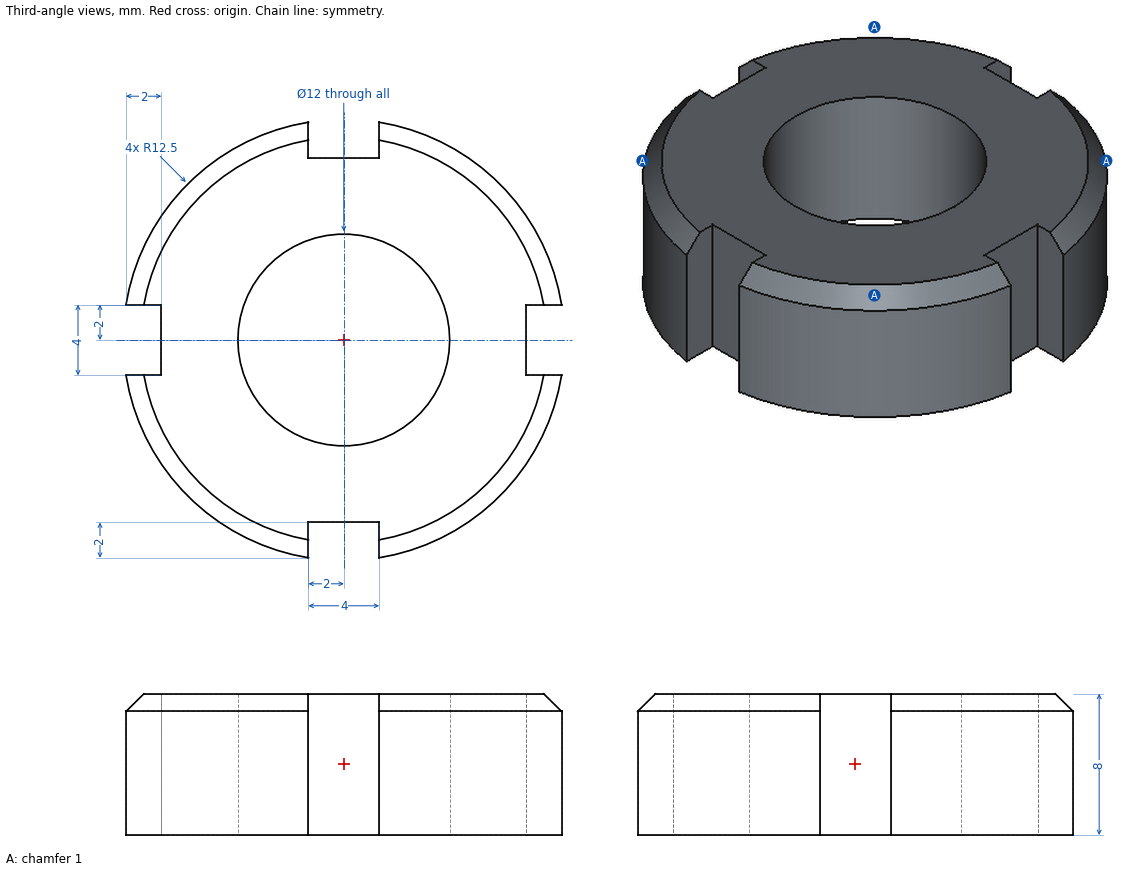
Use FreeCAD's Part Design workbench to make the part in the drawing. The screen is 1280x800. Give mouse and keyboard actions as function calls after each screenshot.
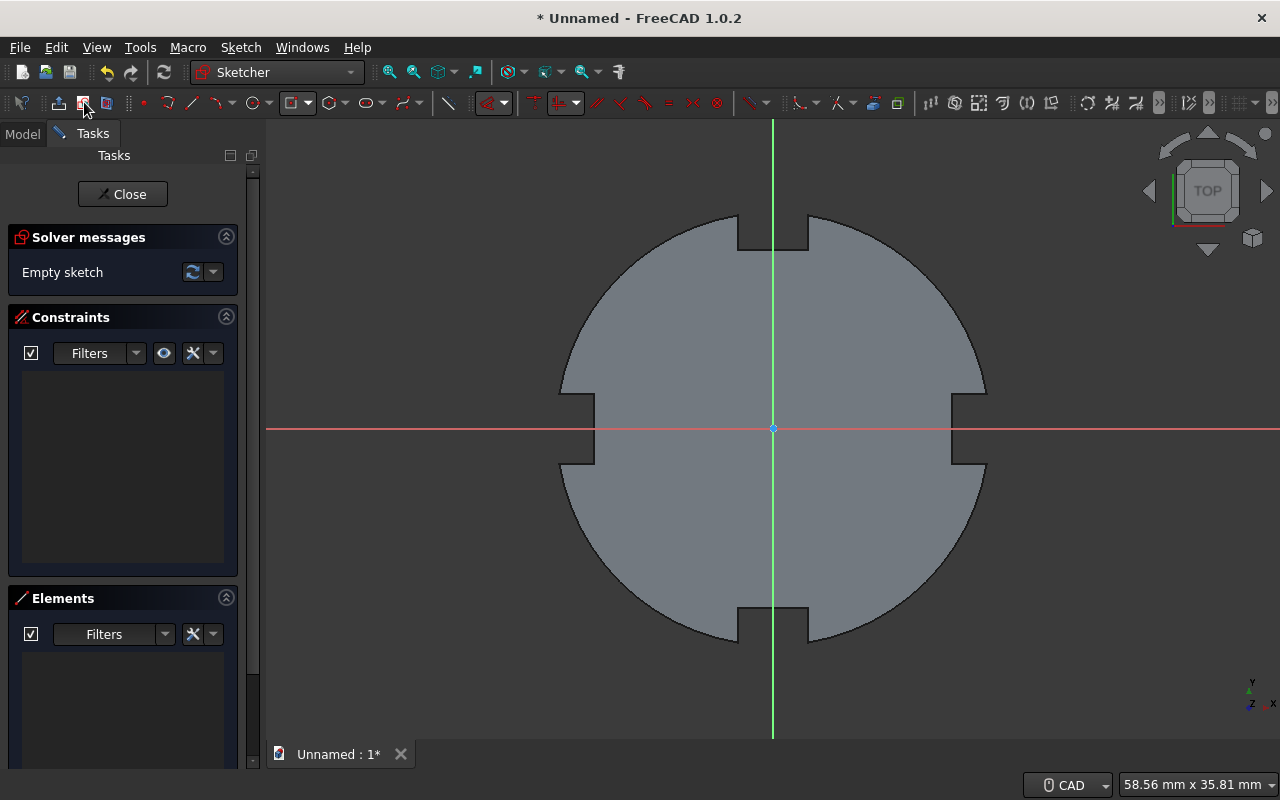
scroll(856, 429, up, 3)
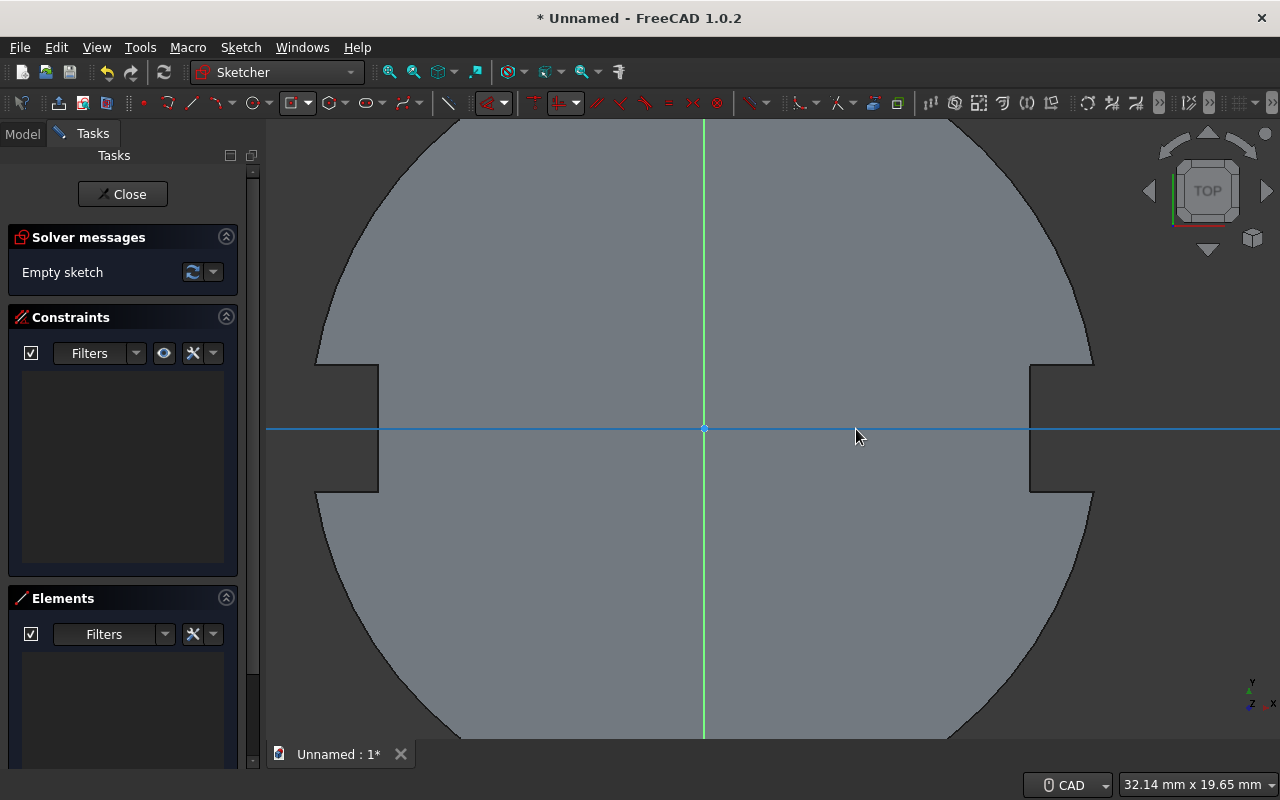
key(g)
key(c)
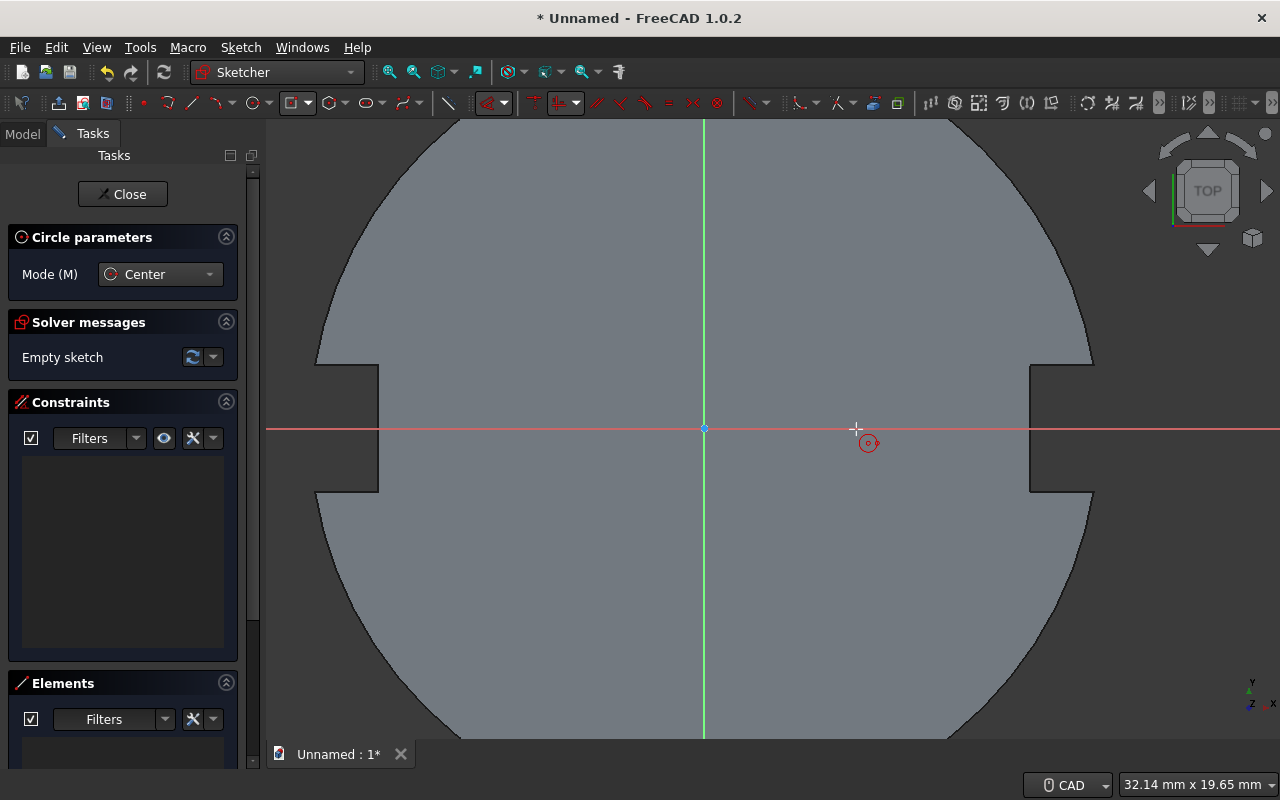
click(704, 429)
click(838, 295)
key(Escape)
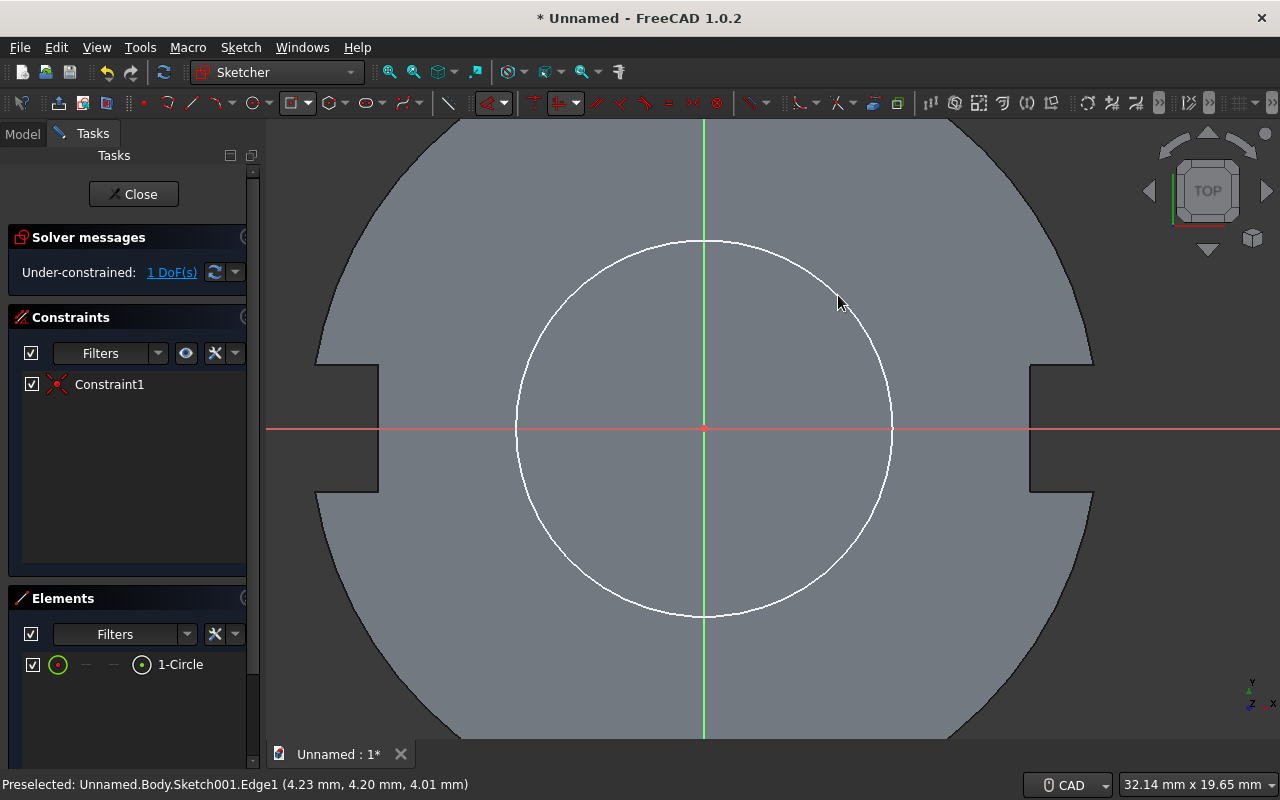
key(d)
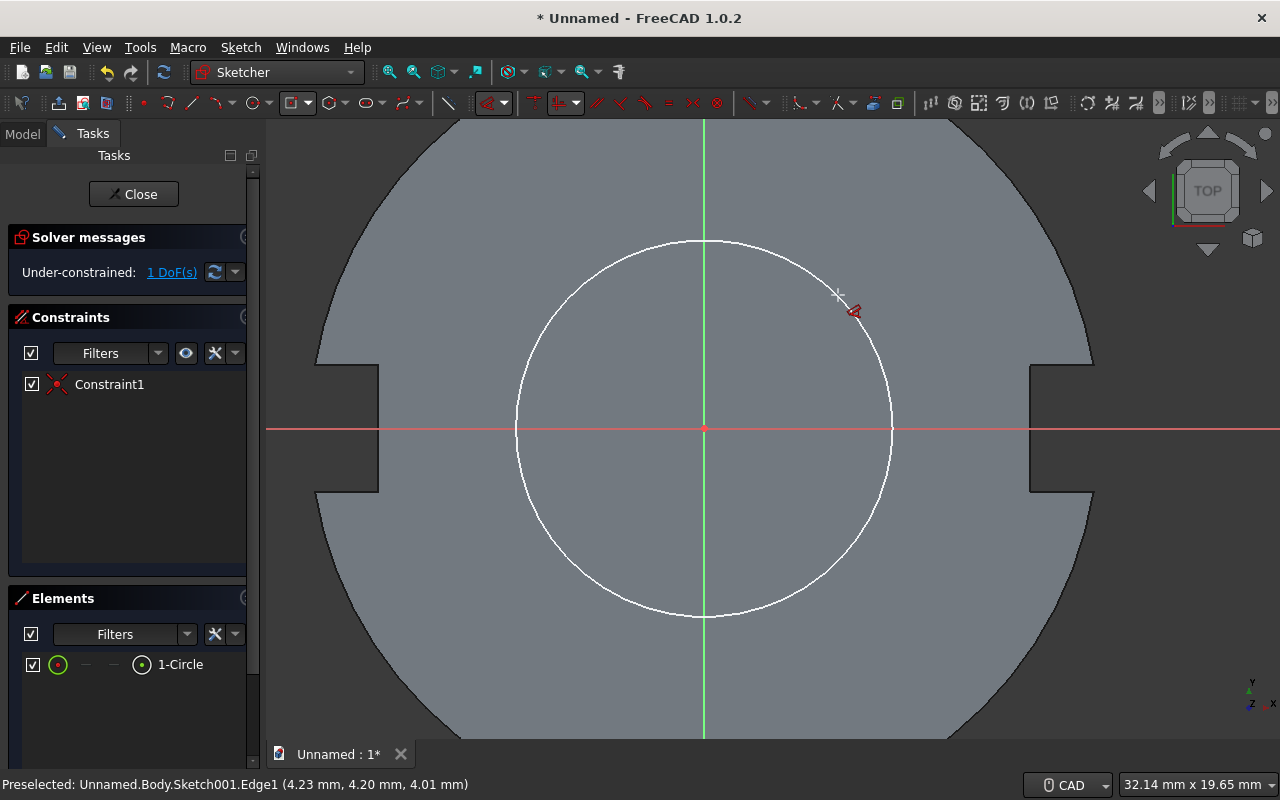
click(837, 295)
click(860, 272)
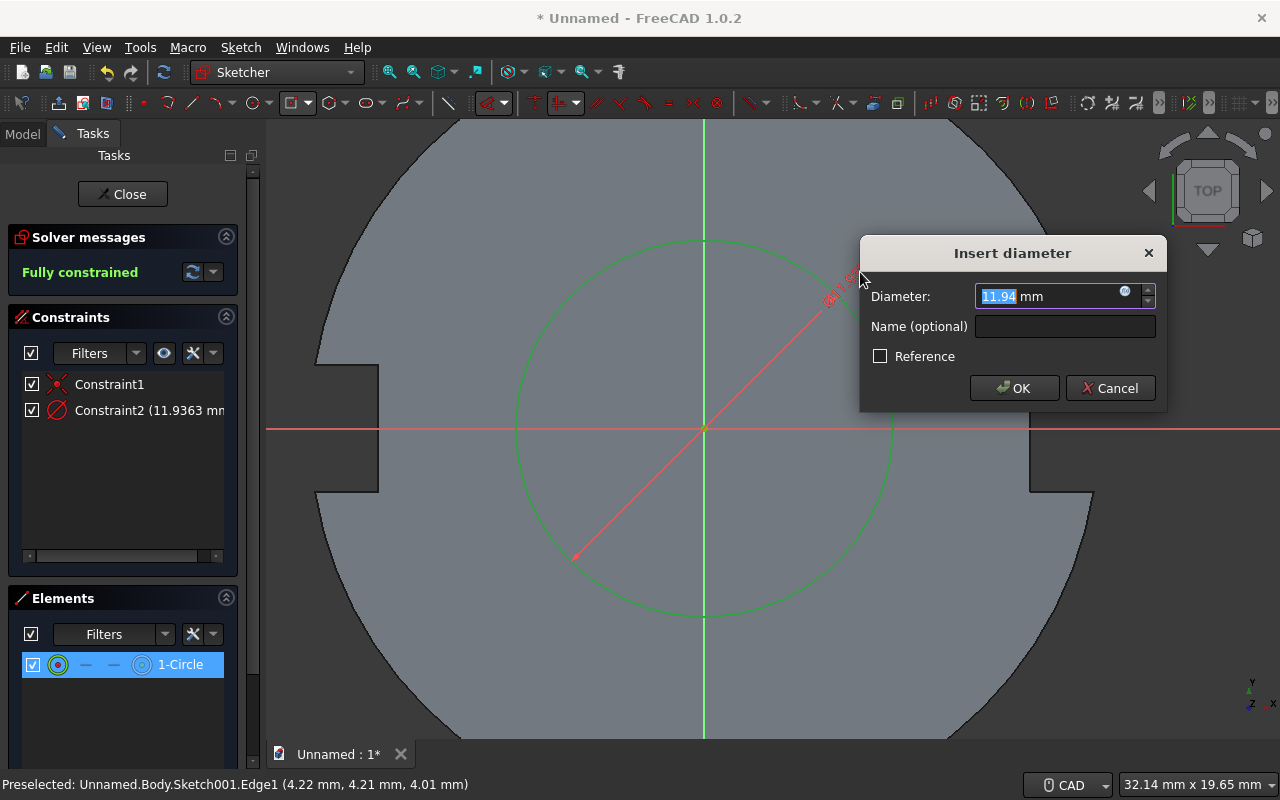
text(12)
key(Return)
key(Escape)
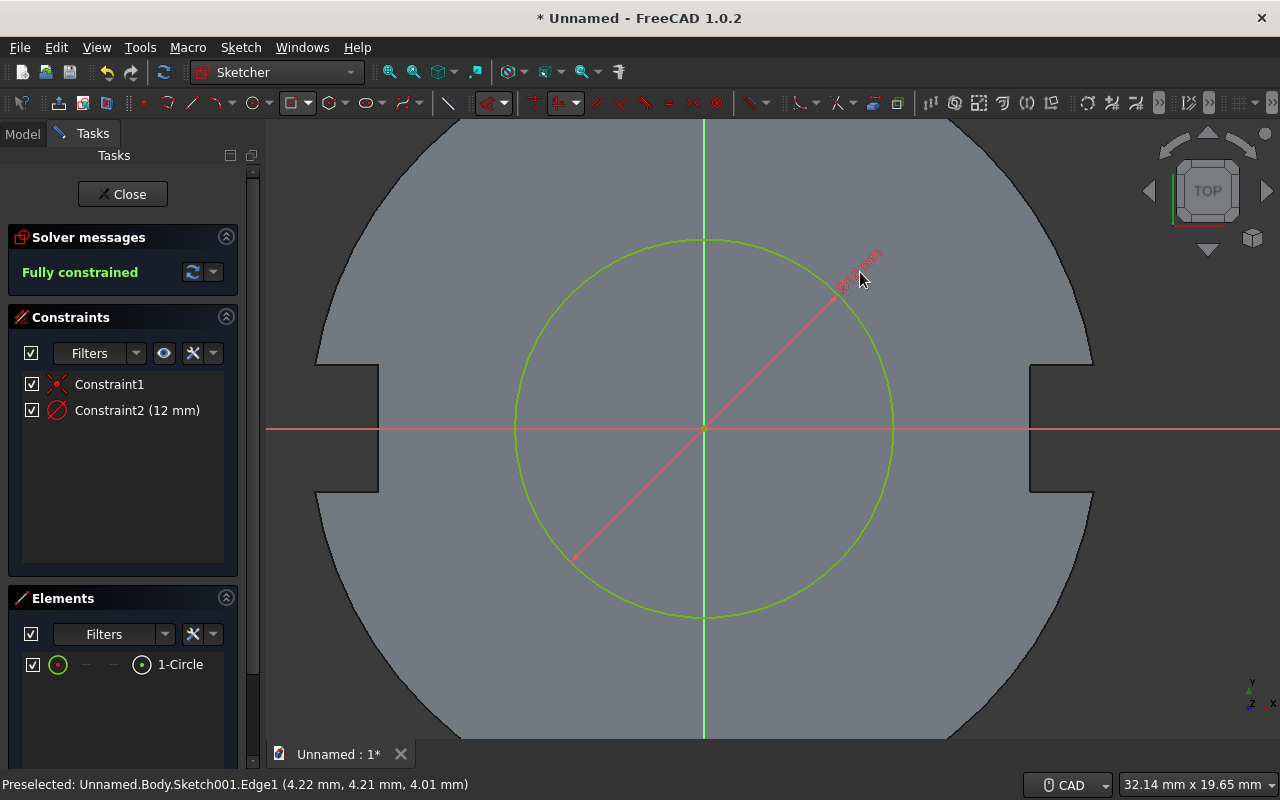
click(123, 194)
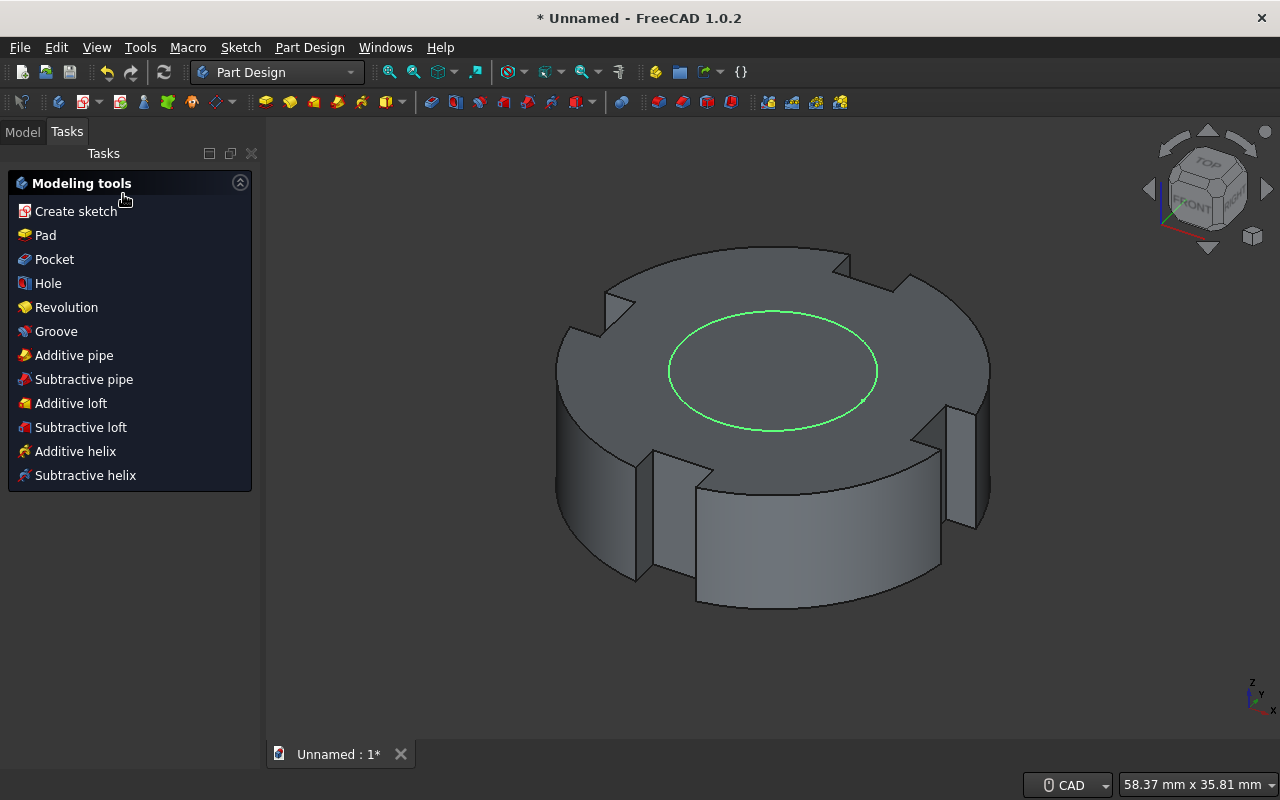
click(456, 102)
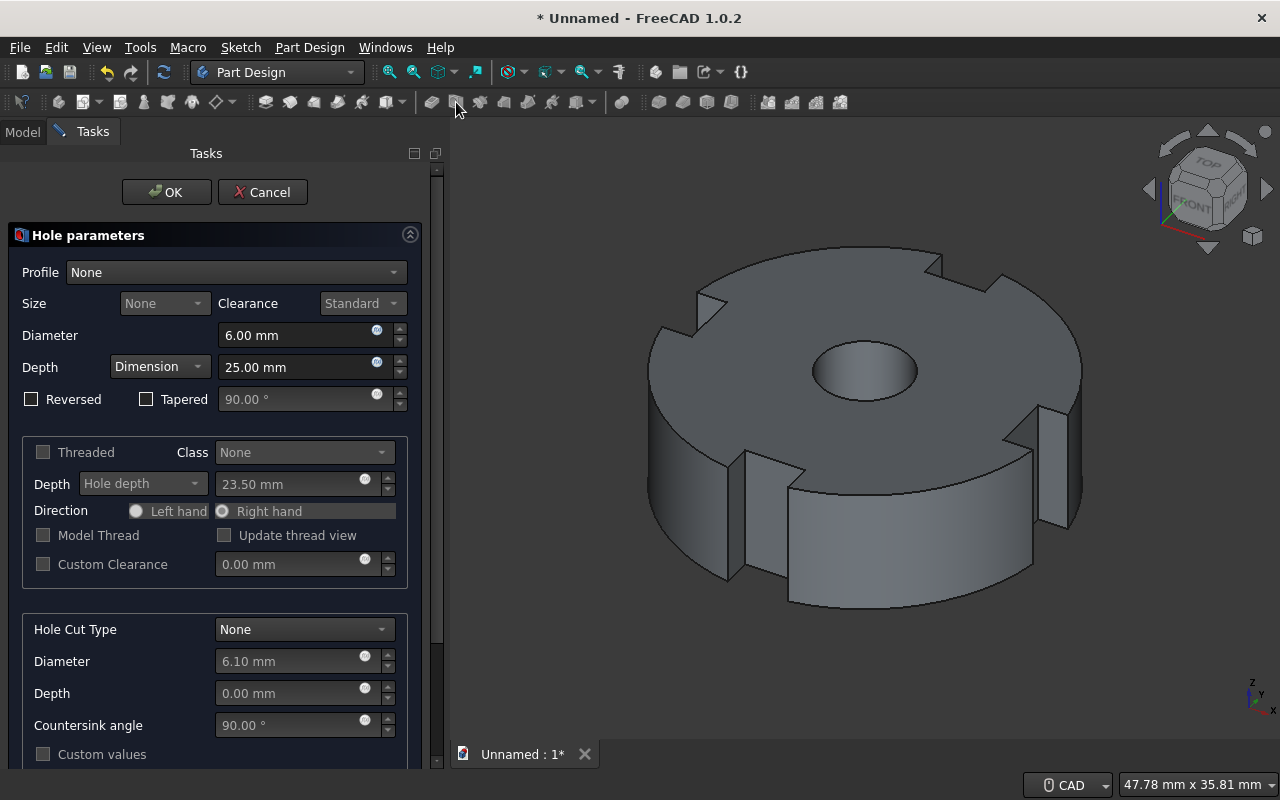
triple_click(305, 335)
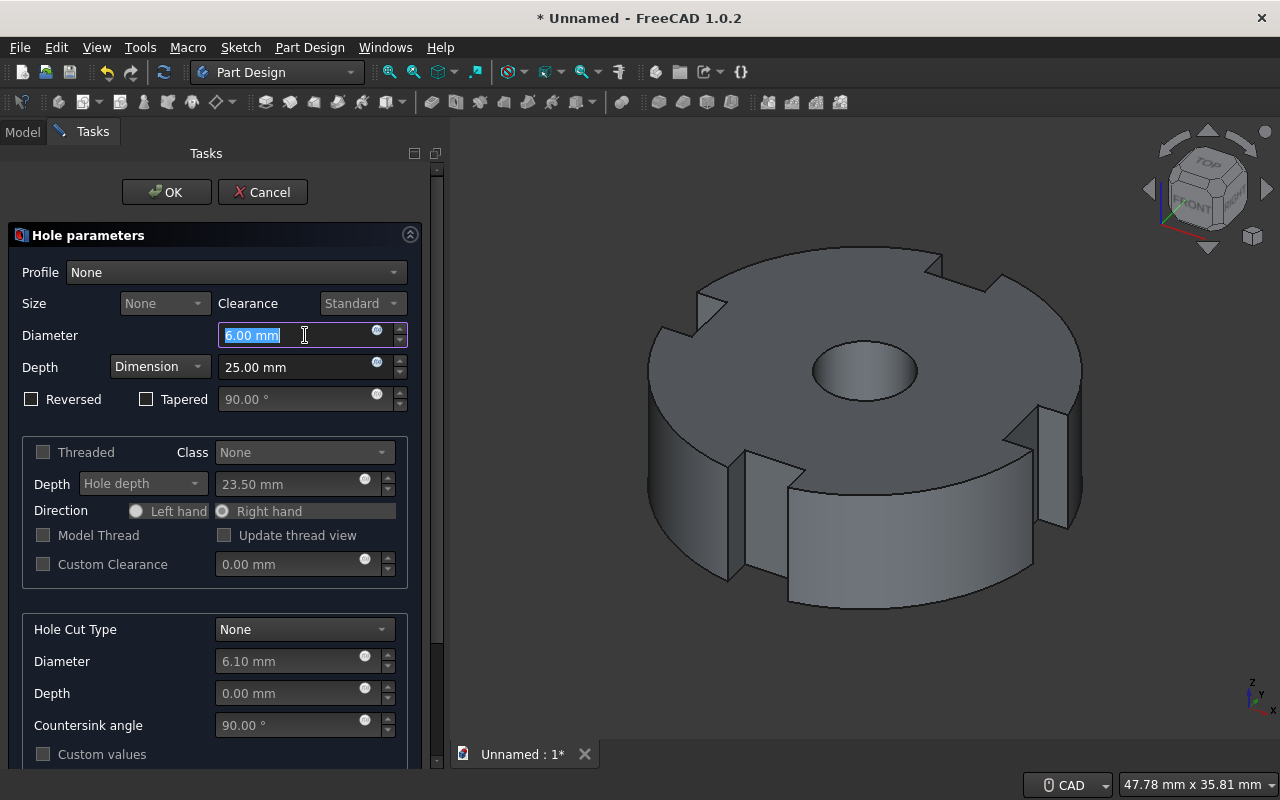
text(12)
key(Tab)